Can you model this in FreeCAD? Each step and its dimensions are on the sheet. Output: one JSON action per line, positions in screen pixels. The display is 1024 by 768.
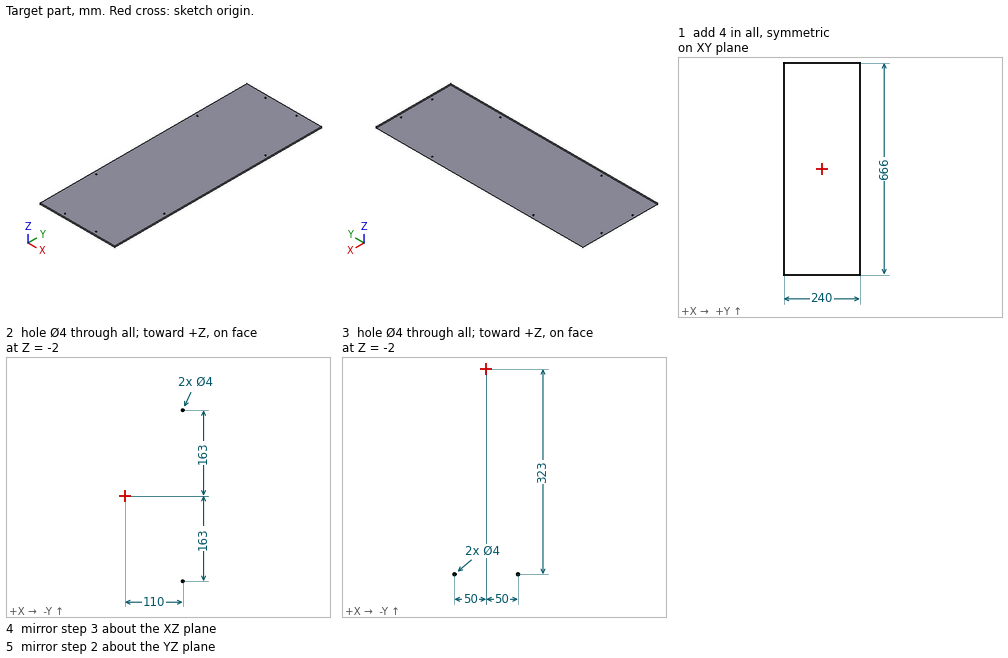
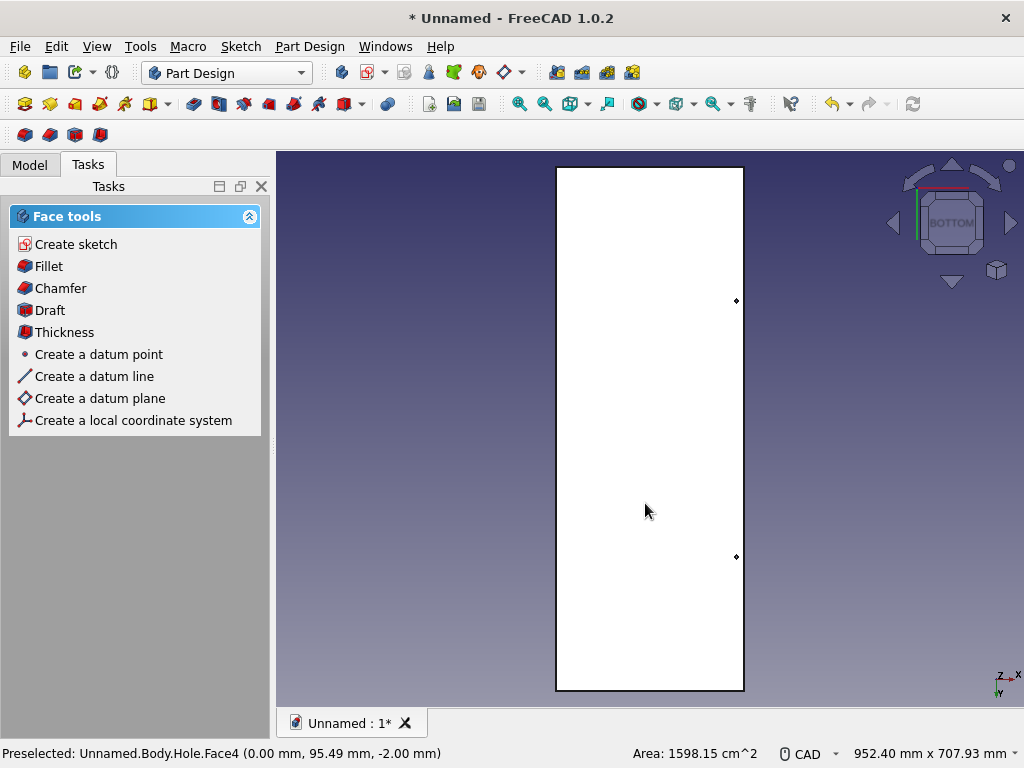
{"action": "left_click", "coordinate": [366, 72]}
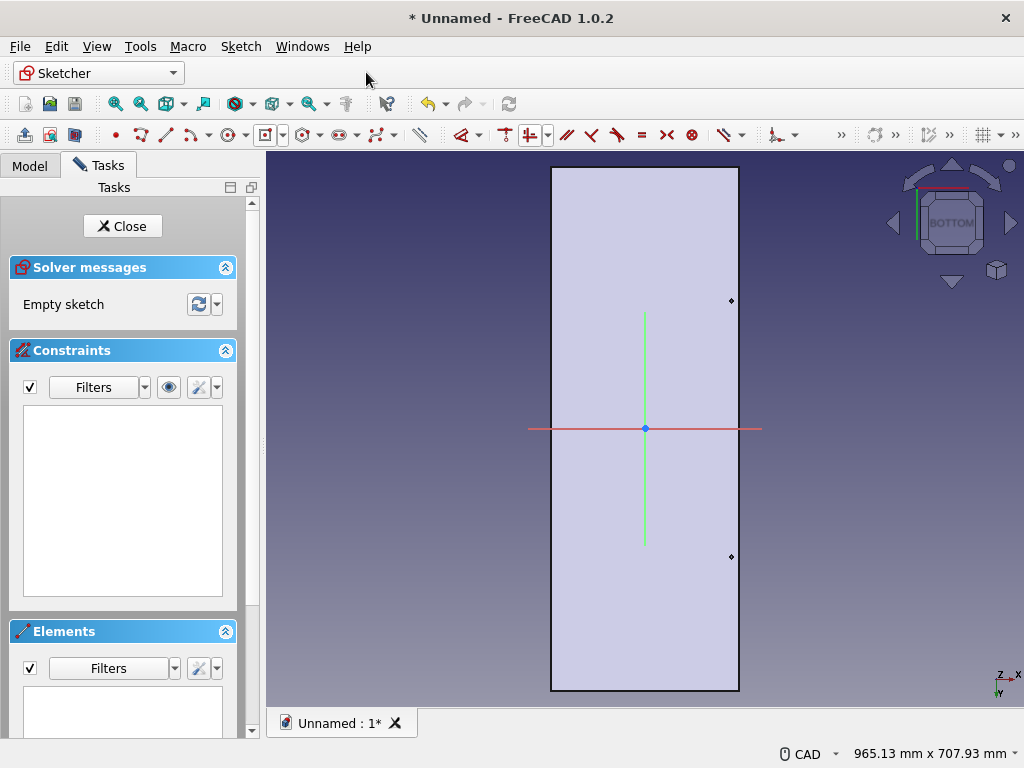
{"action": "scroll", "coordinate": [576, 429], "scroll_direction": "down", "scroll_amount": 5}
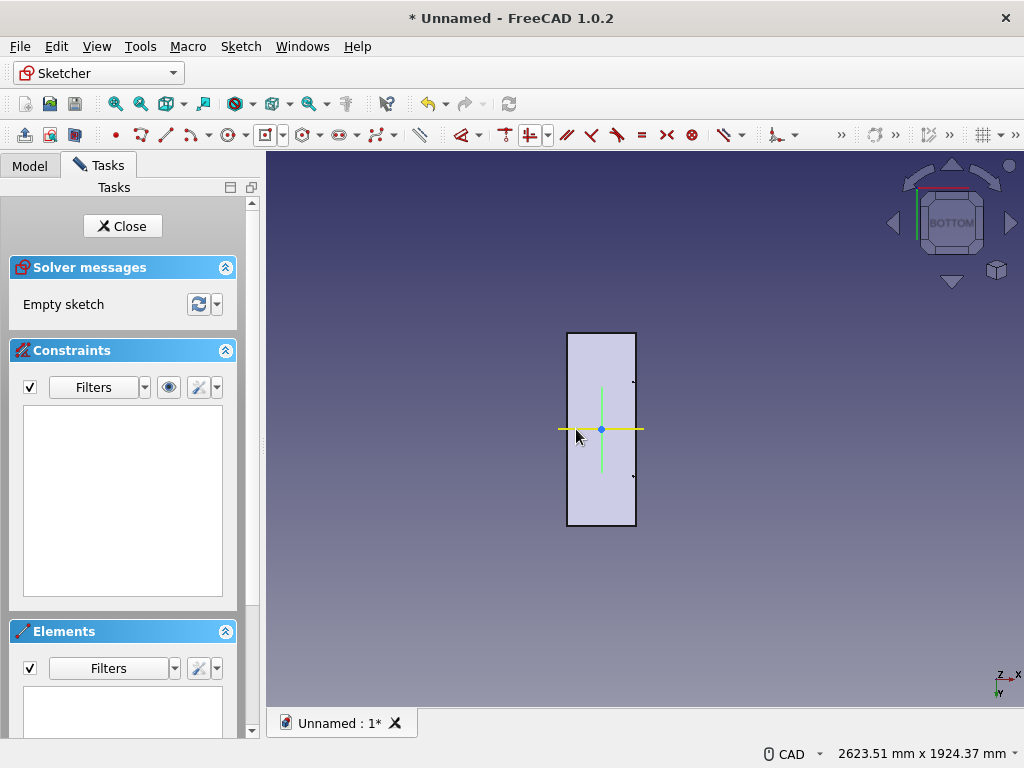
{"action": "scroll", "coordinate": [604, 530], "scroll_direction": "up", "scroll_amount": 13}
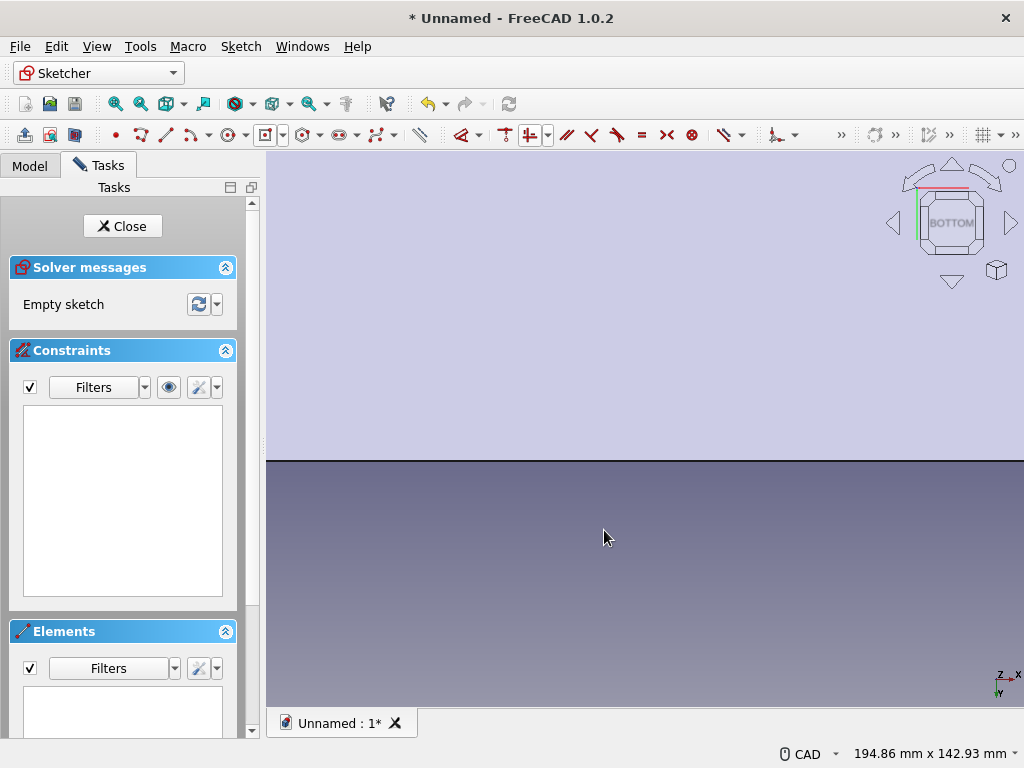
{"action": "left_click", "coordinate": [228, 136]}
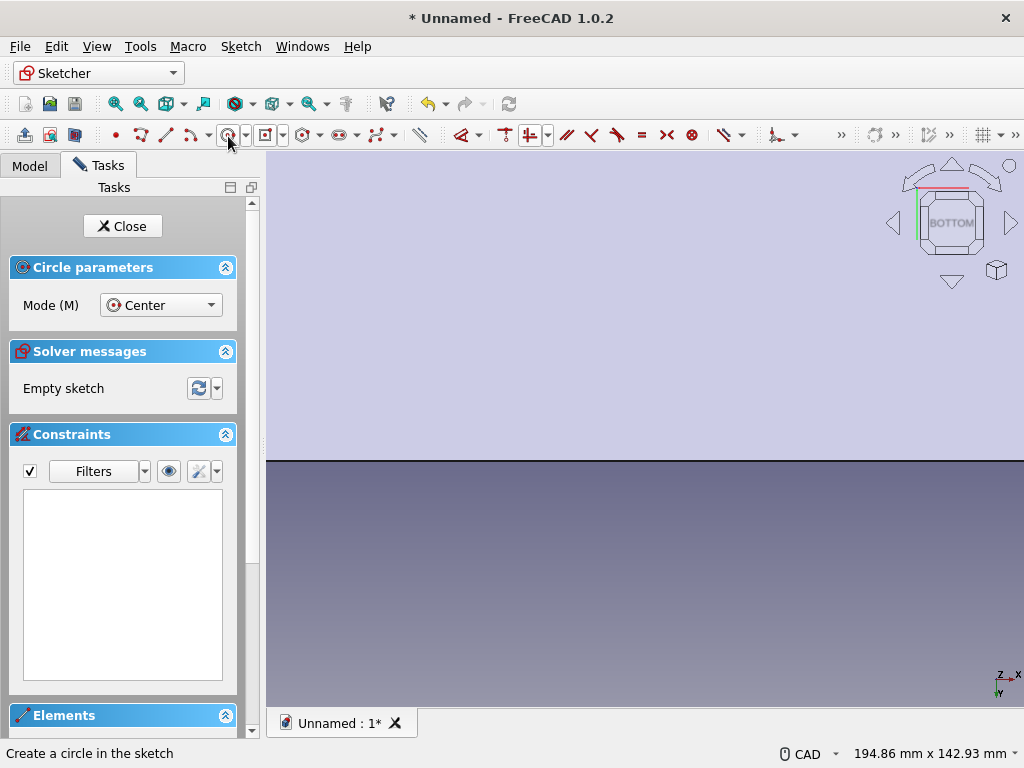
{"action": "scroll", "coordinate": [761, 422], "scroll_direction": "up", "scroll_amount": 6}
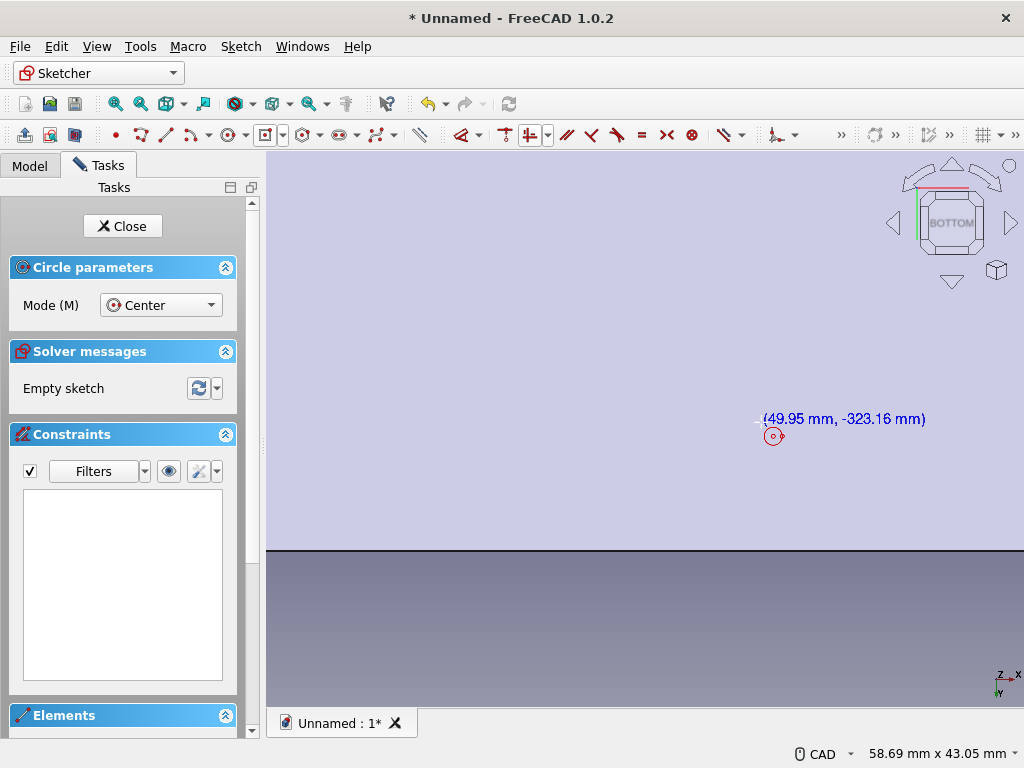
{"action": "left_click", "coordinate": [760, 422]}
{"action": "left_click", "coordinate": [778, 404]}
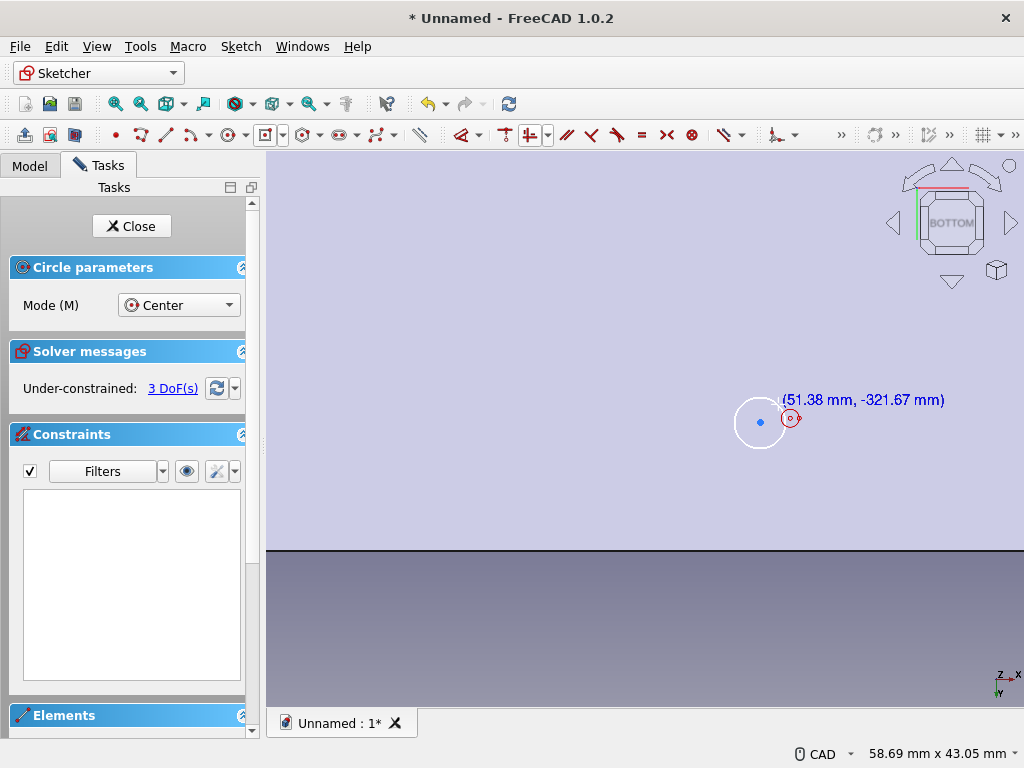
{"action": "scroll", "coordinate": [776, 432], "scroll_direction": "down", "scroll_amount": 6}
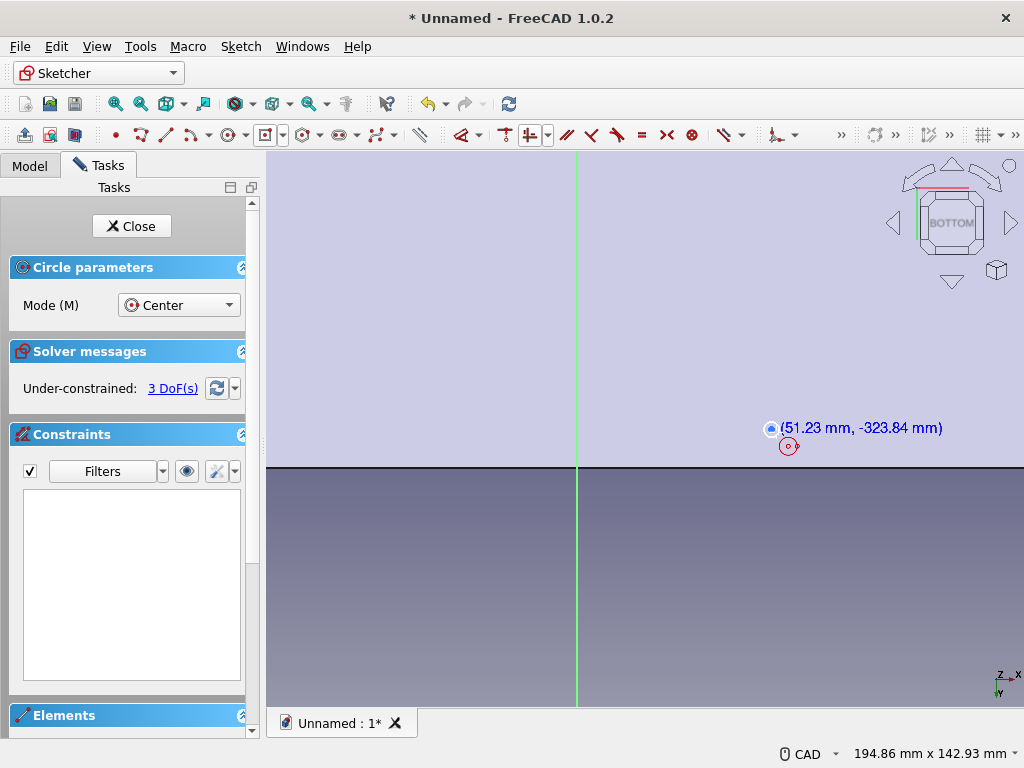
{"action": "scroll", "coordinate": [383, 429], "scroll_direction": "up", "scroll_amount": 6}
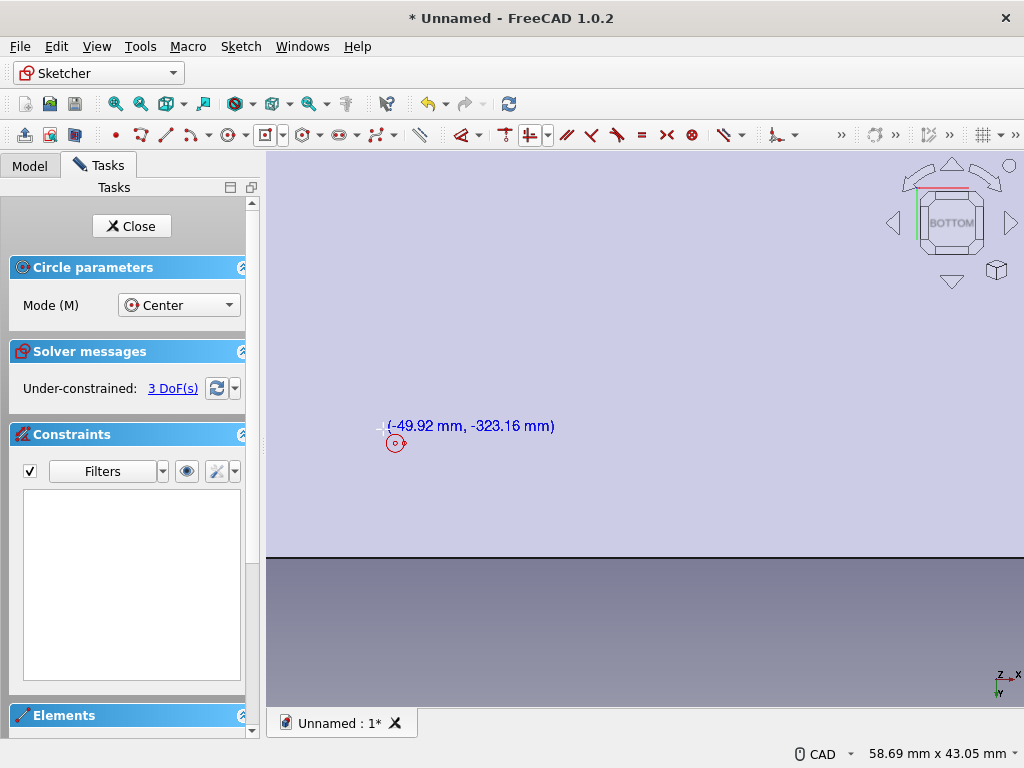
{"action": "left_click", "coordinate": [382, 429]}
{"action": "left_click", "coordinate": [400, 411]}
{"action": "key", "text": "Escape"}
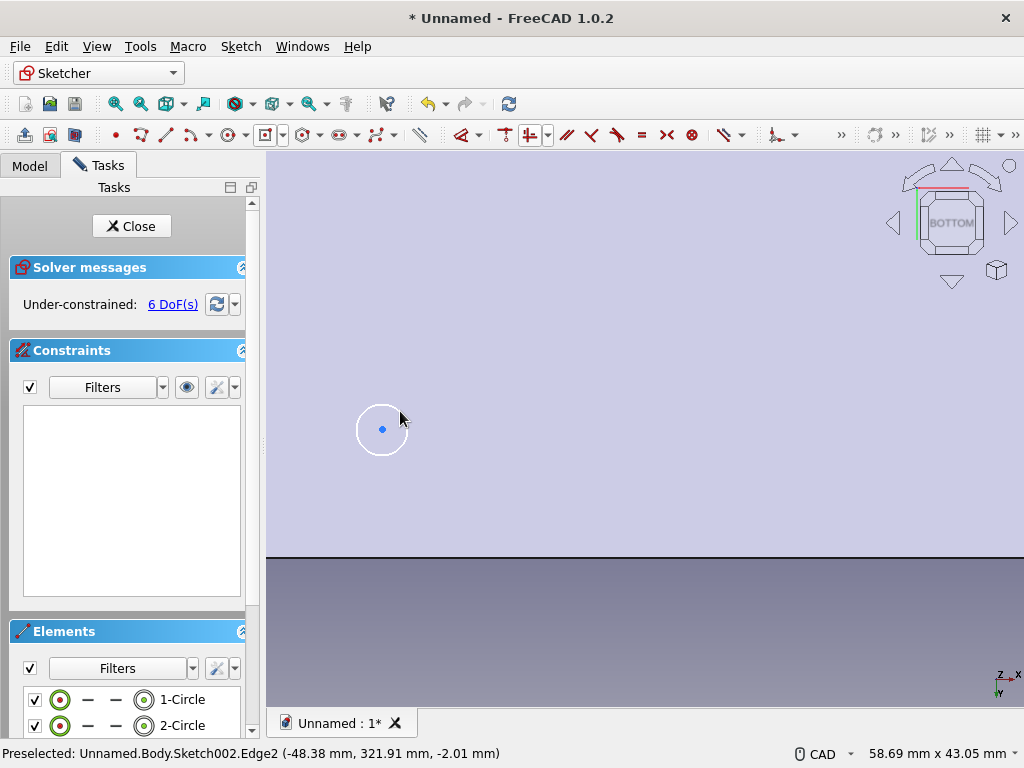
{"action": "scroll", "coordinate": [382, 429], "scroll_direction": "down", "scroll_amount": 6}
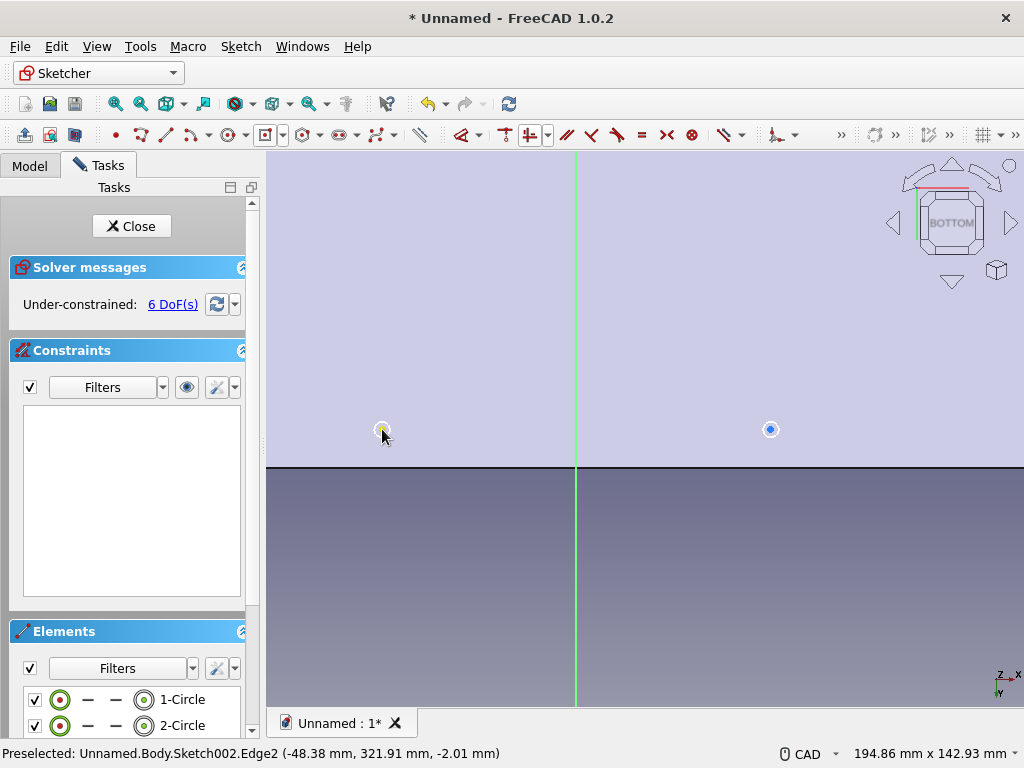
{"action": "scroll", "coordinate": [776, 424], "scroll_direction": "up", "scroll_amount": 3}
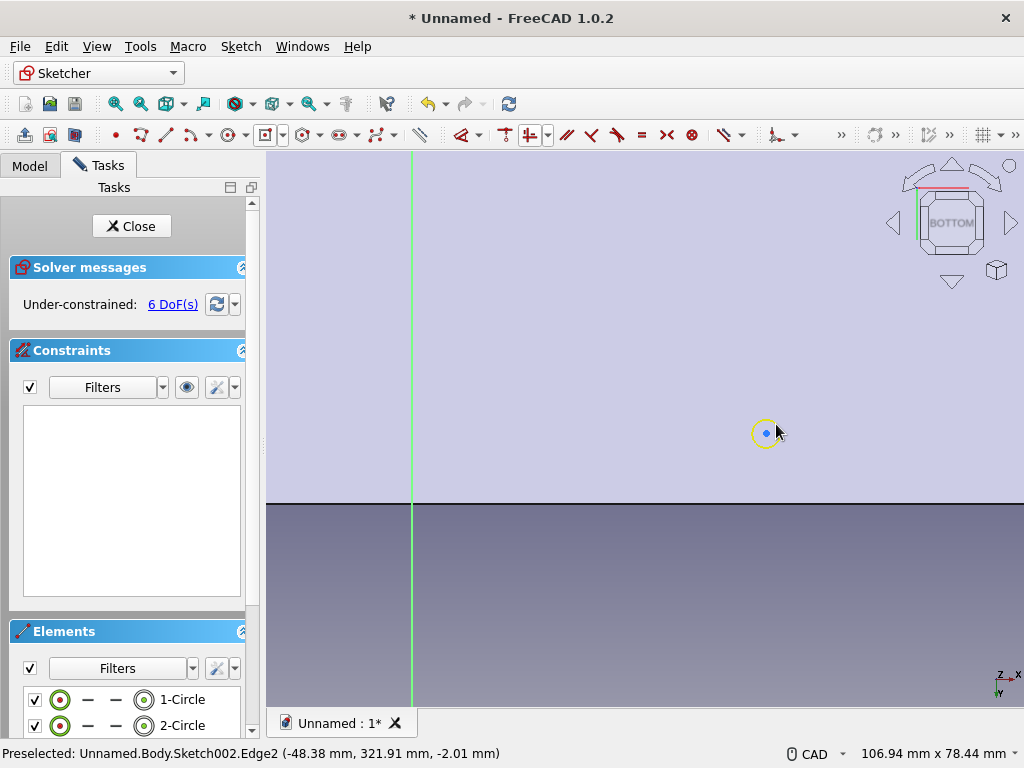
{"action": "left_click", "coordinate": [776, 424]}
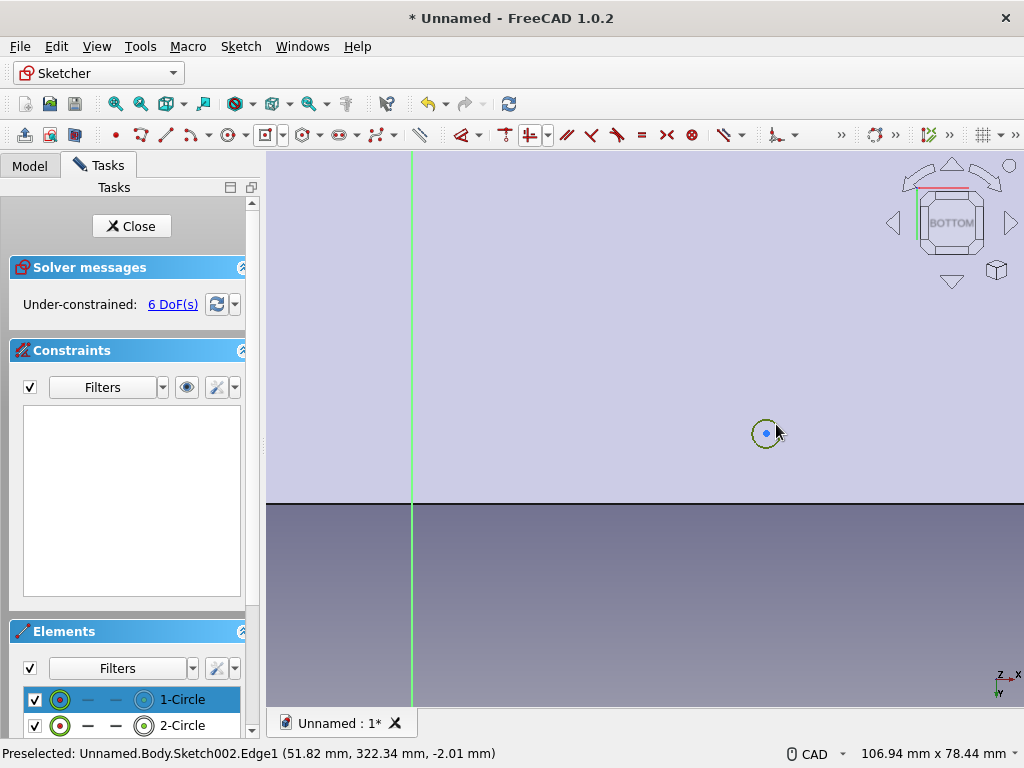
{"action": "scroll", "coordinate": [777, 424], "scroll_direction": "down", "scroll_amount": 3}